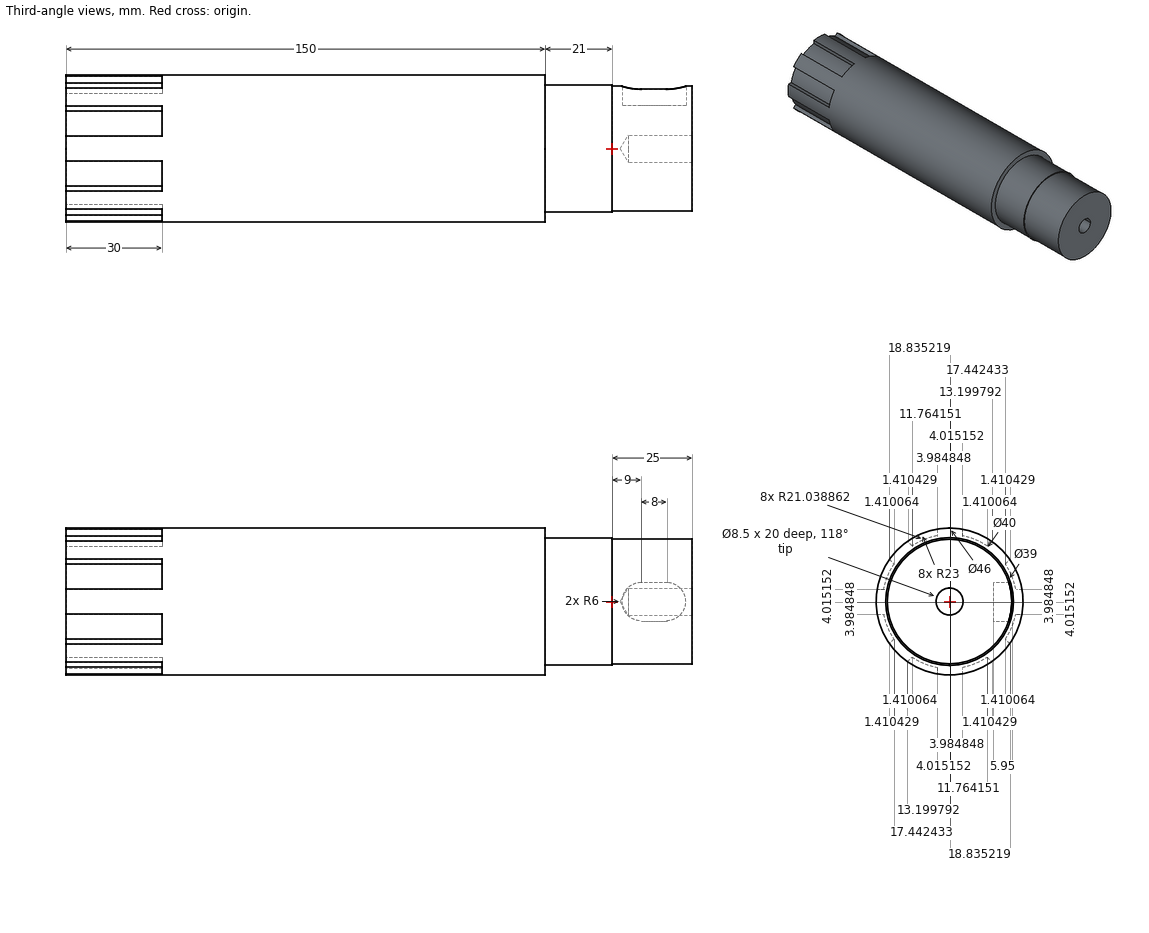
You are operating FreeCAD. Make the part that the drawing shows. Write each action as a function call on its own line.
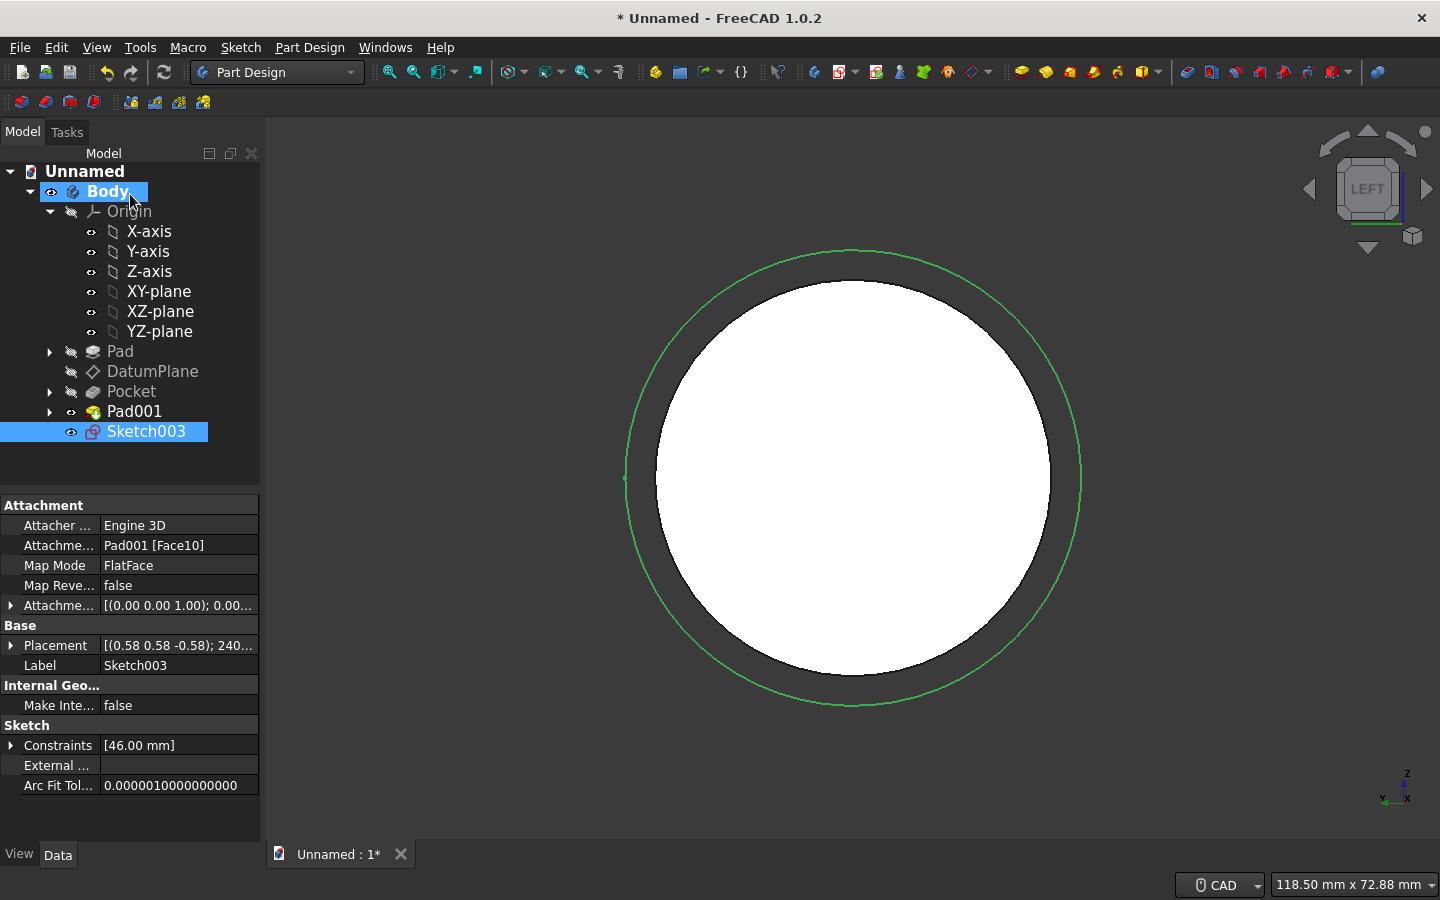
click(1022, 72)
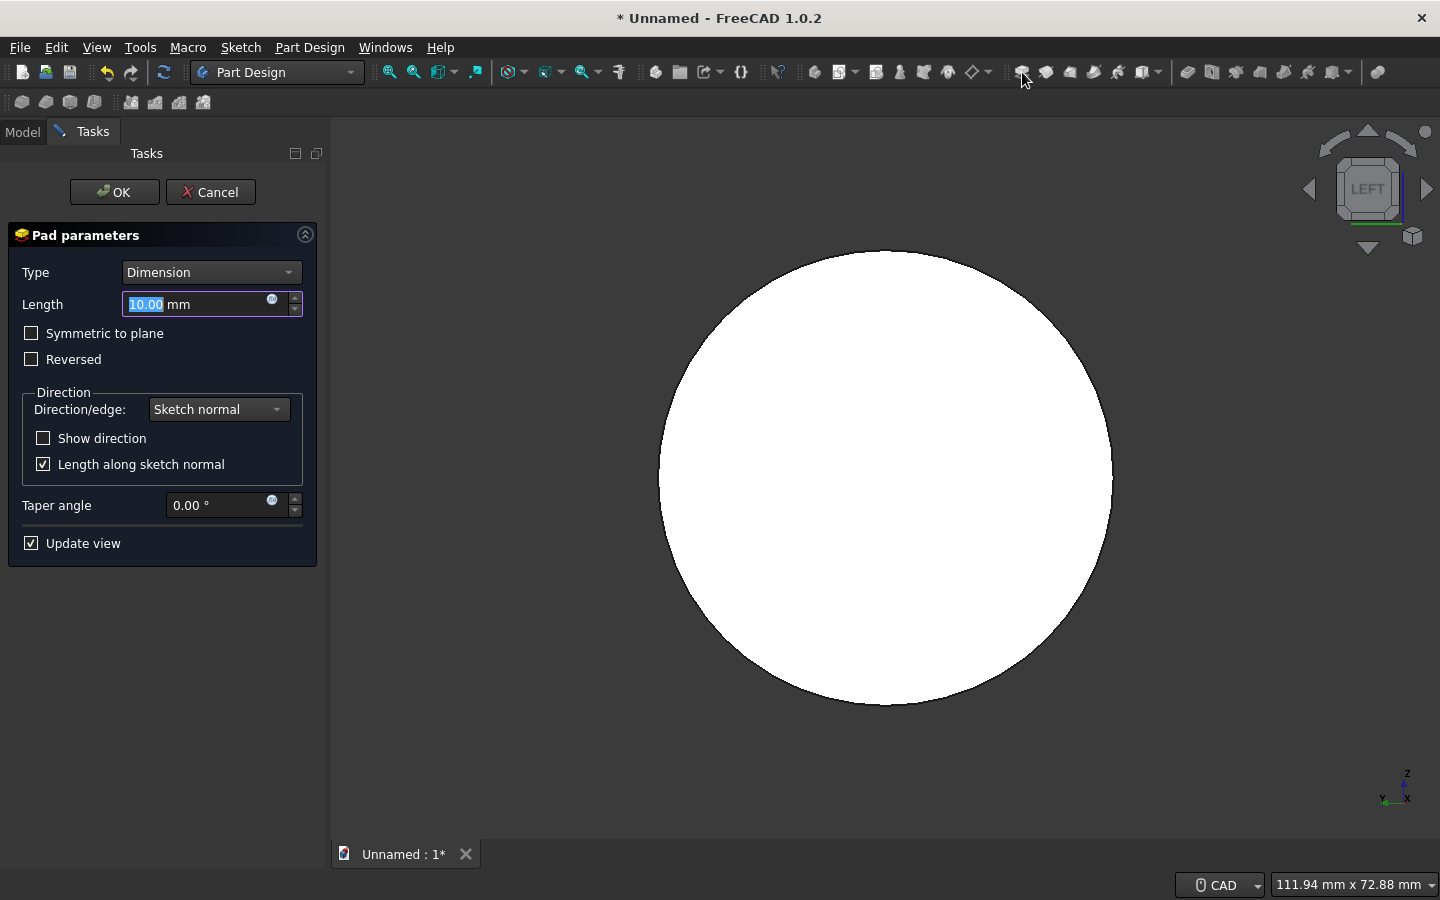
text(150)
key(Tab)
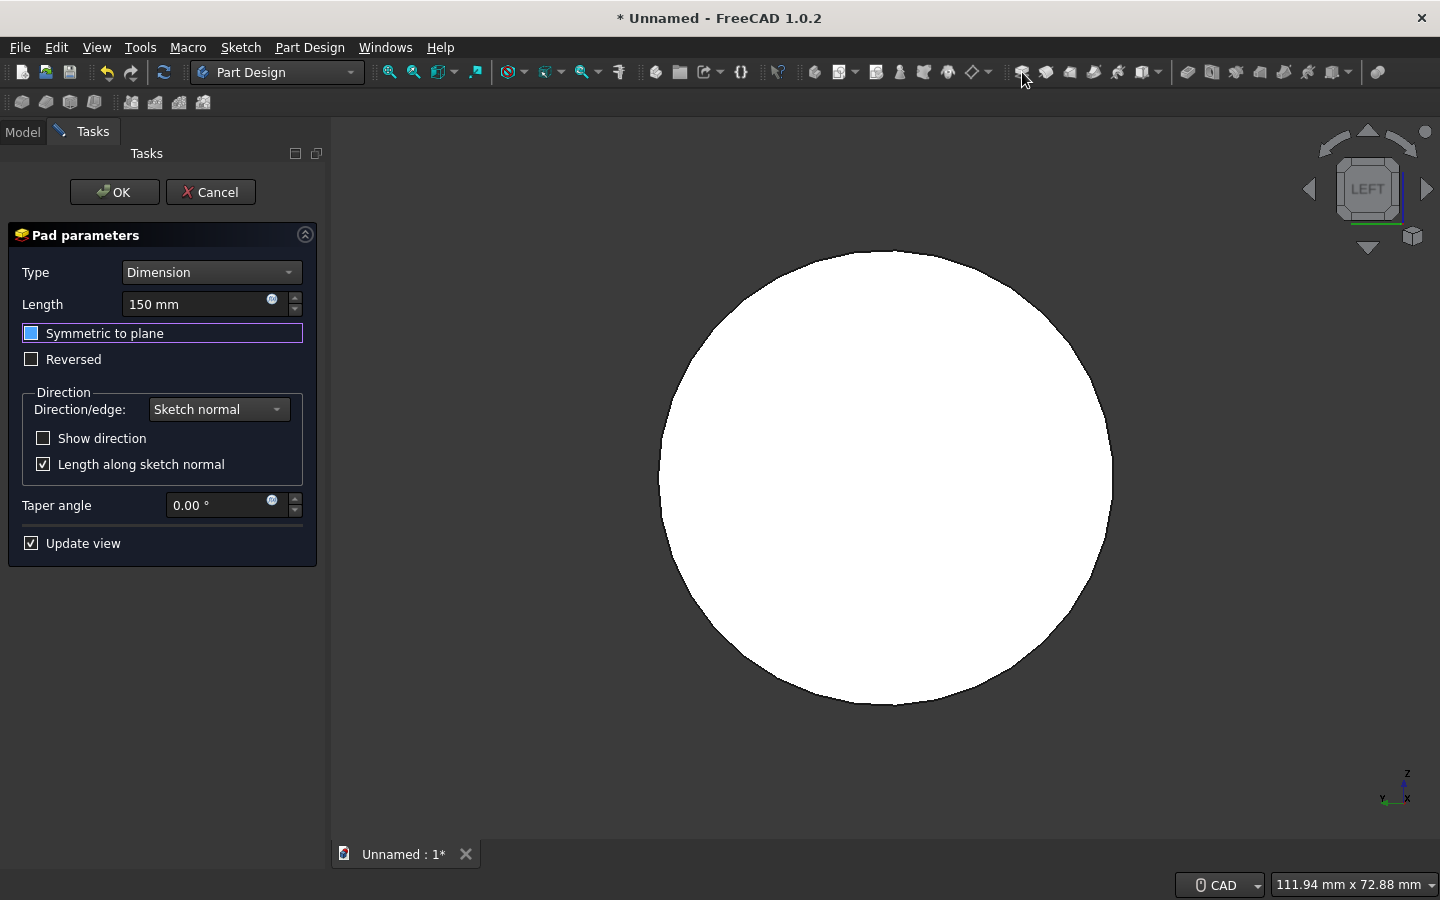
click(115, 192)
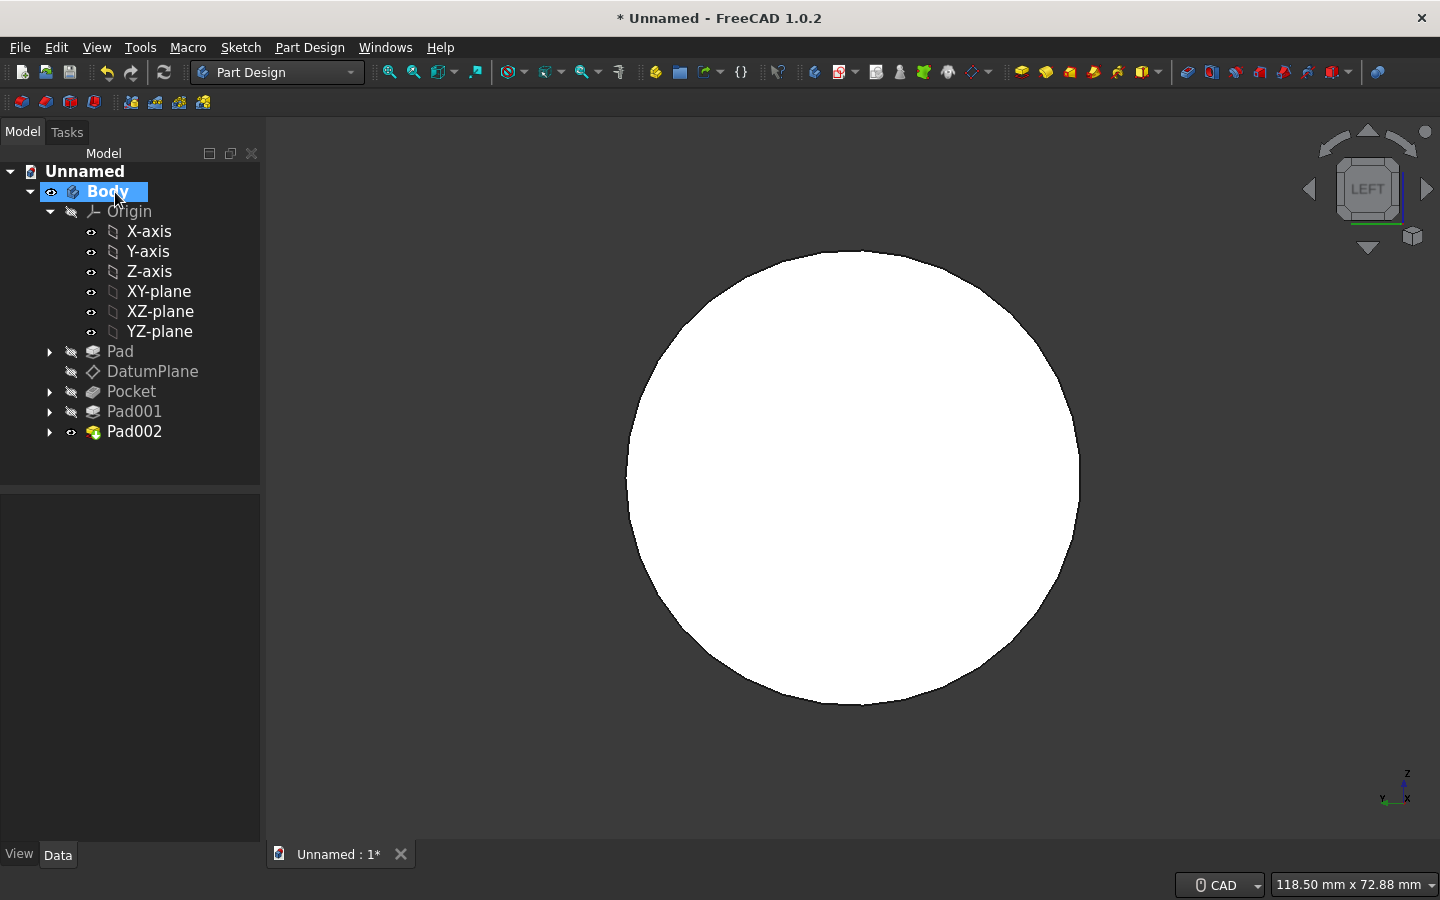
click(136, 332)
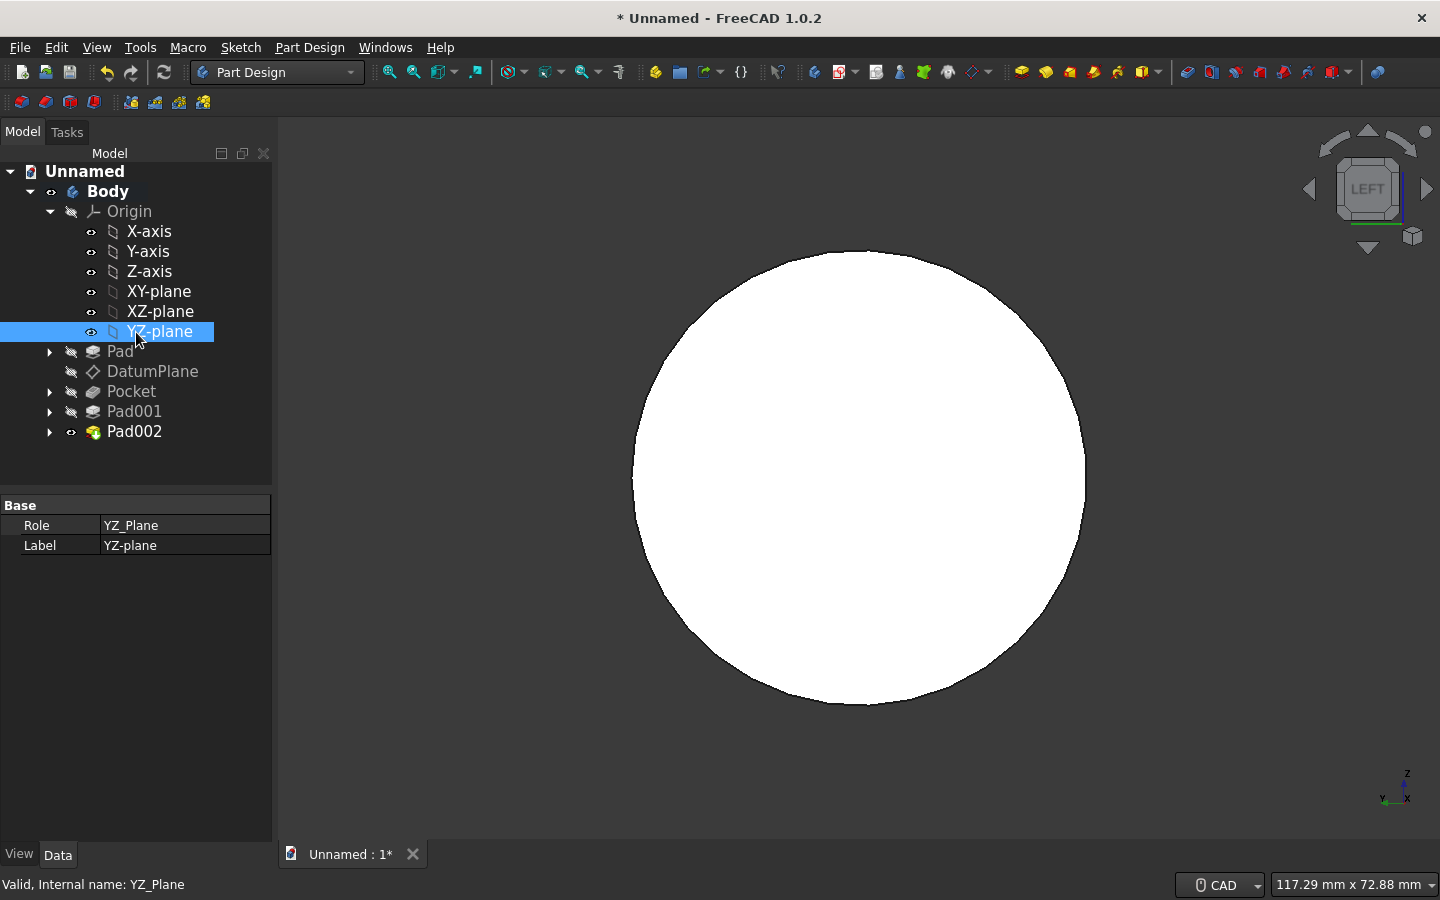
click(972, 72)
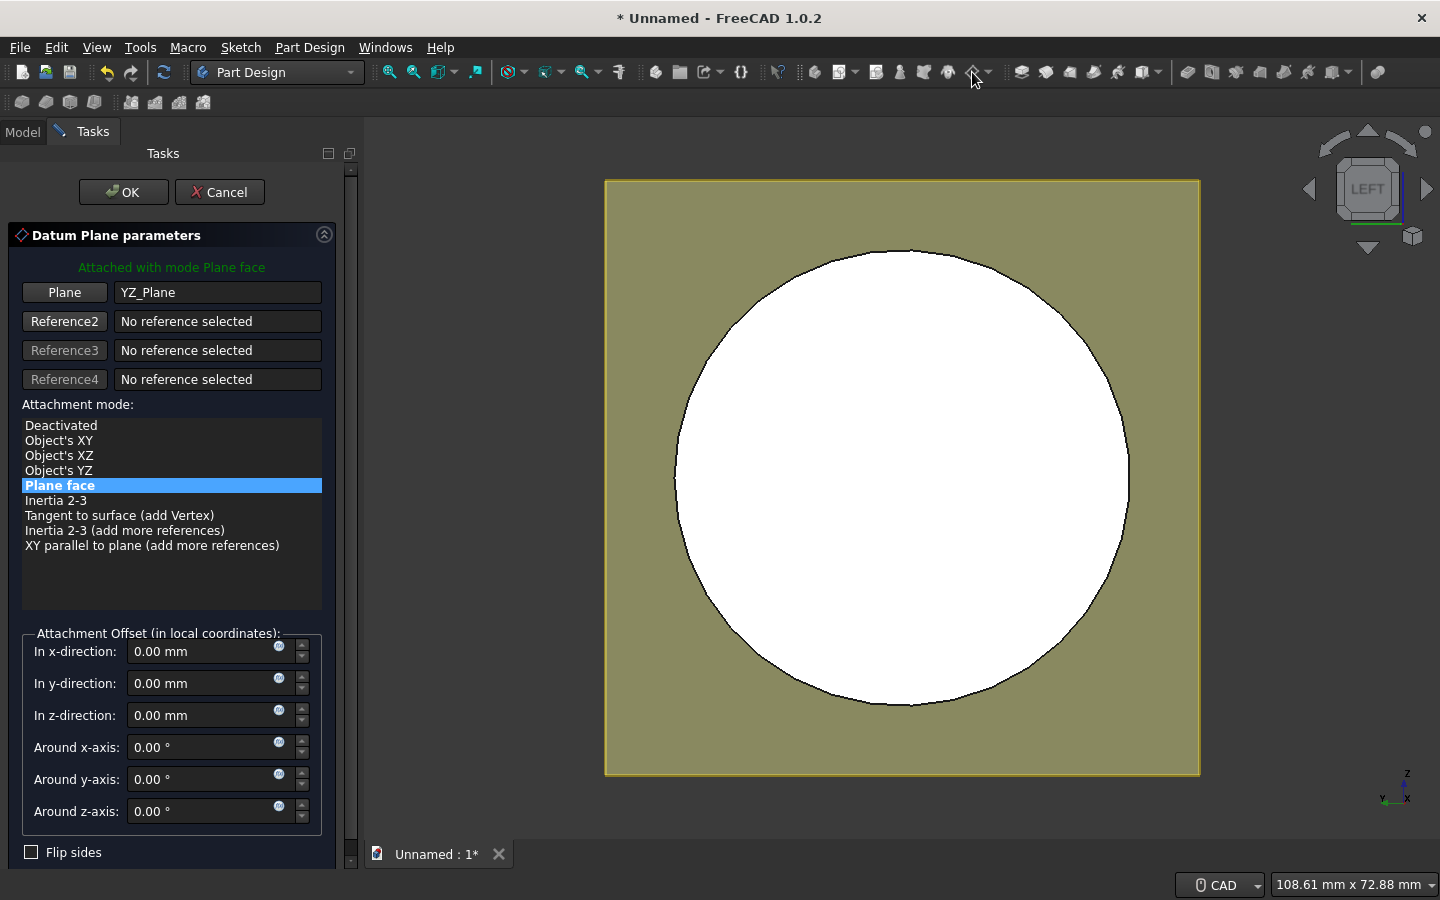
triple_click(210, 715)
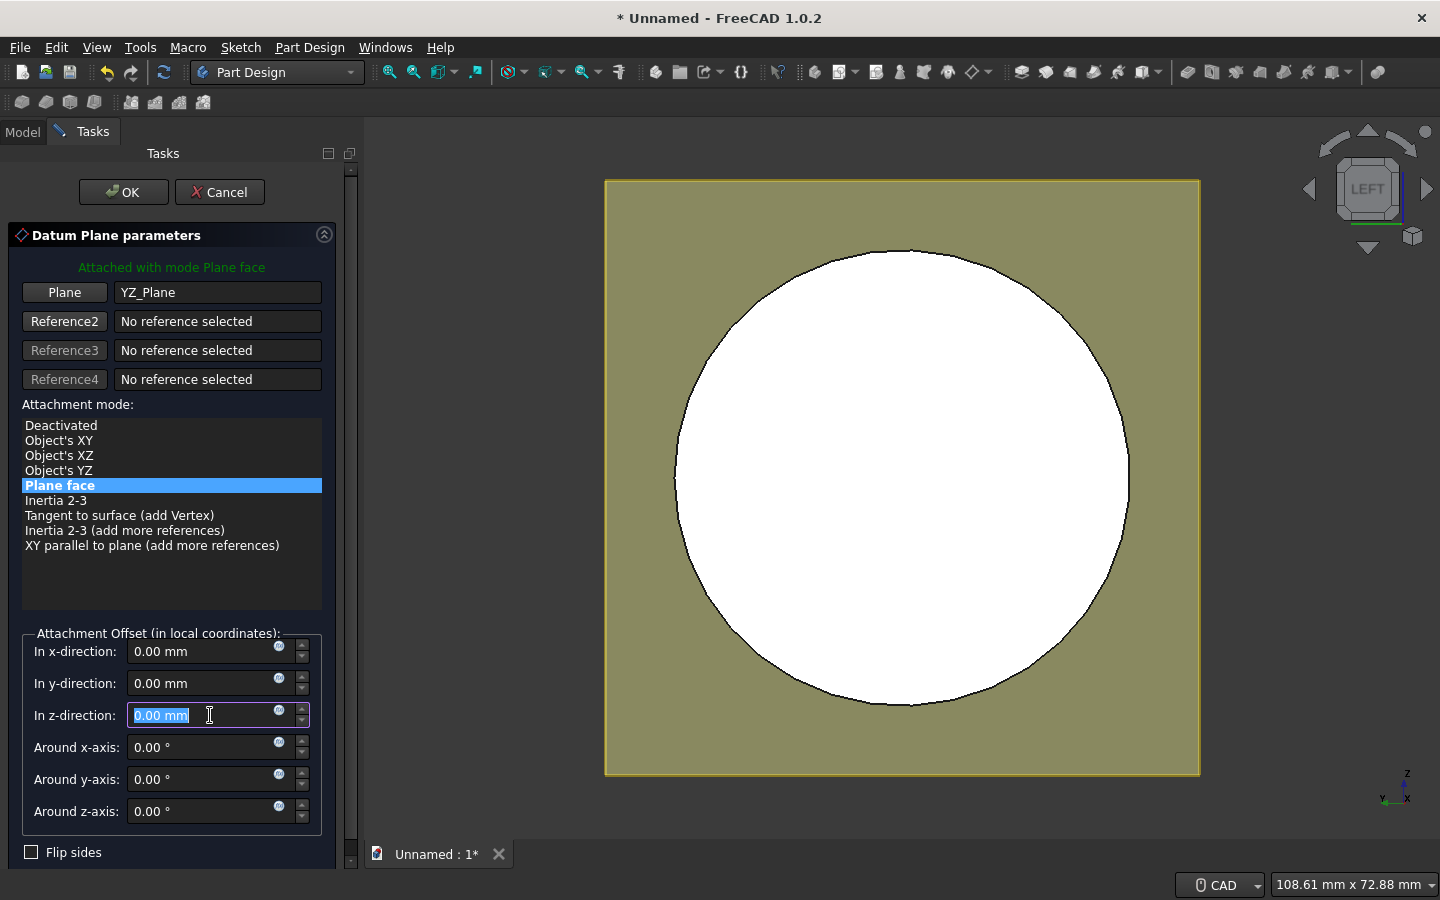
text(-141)
key(Tab)